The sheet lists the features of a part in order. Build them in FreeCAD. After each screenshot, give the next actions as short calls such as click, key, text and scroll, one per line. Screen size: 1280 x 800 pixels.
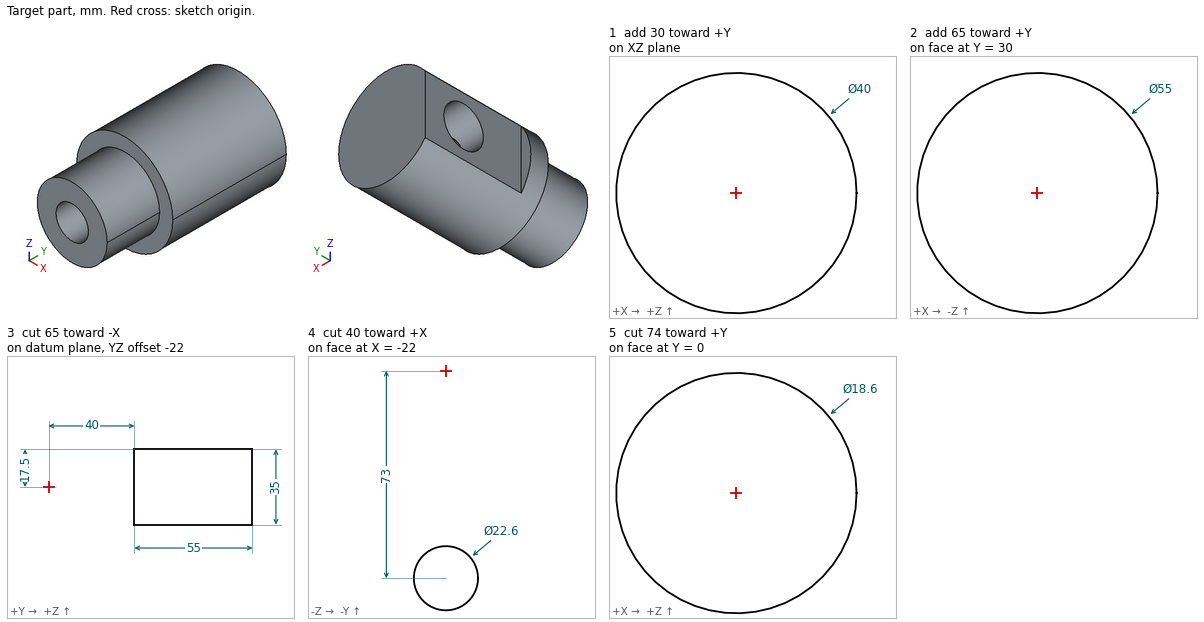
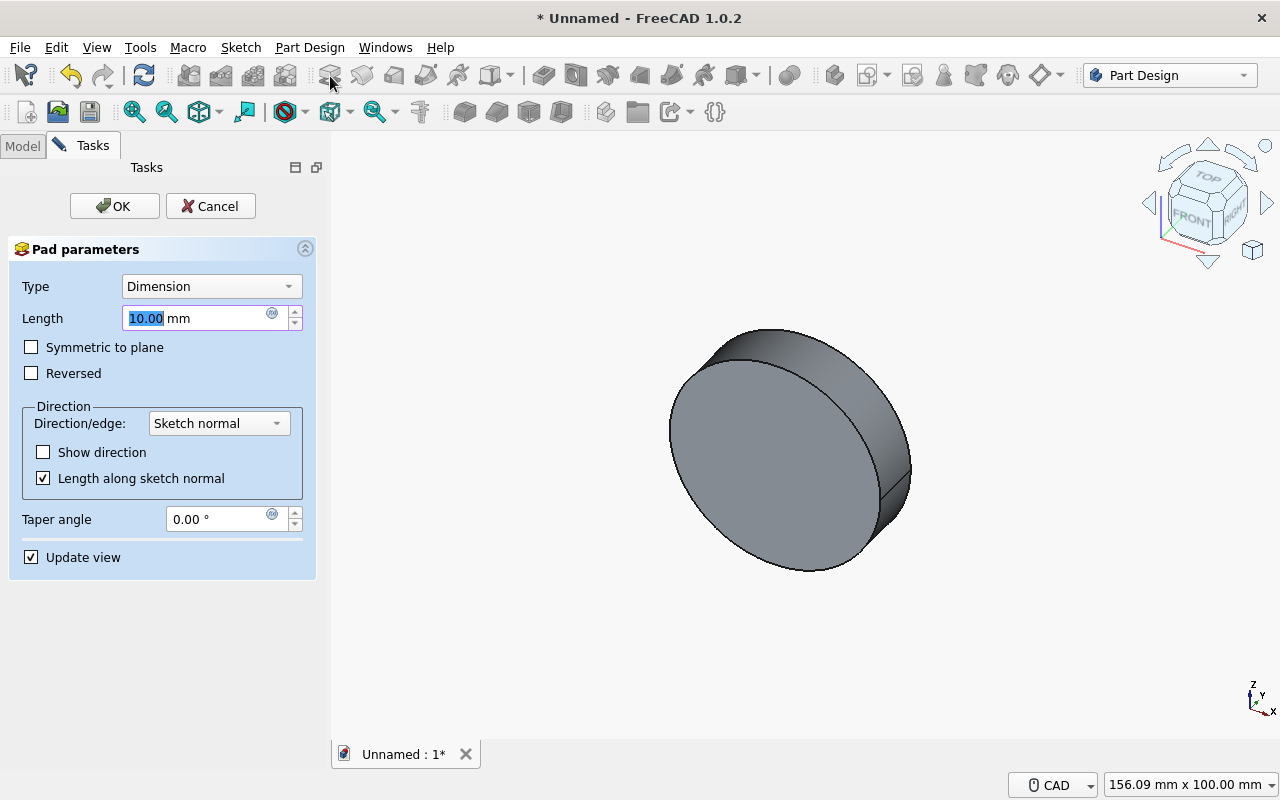
text(30)
key(Tab)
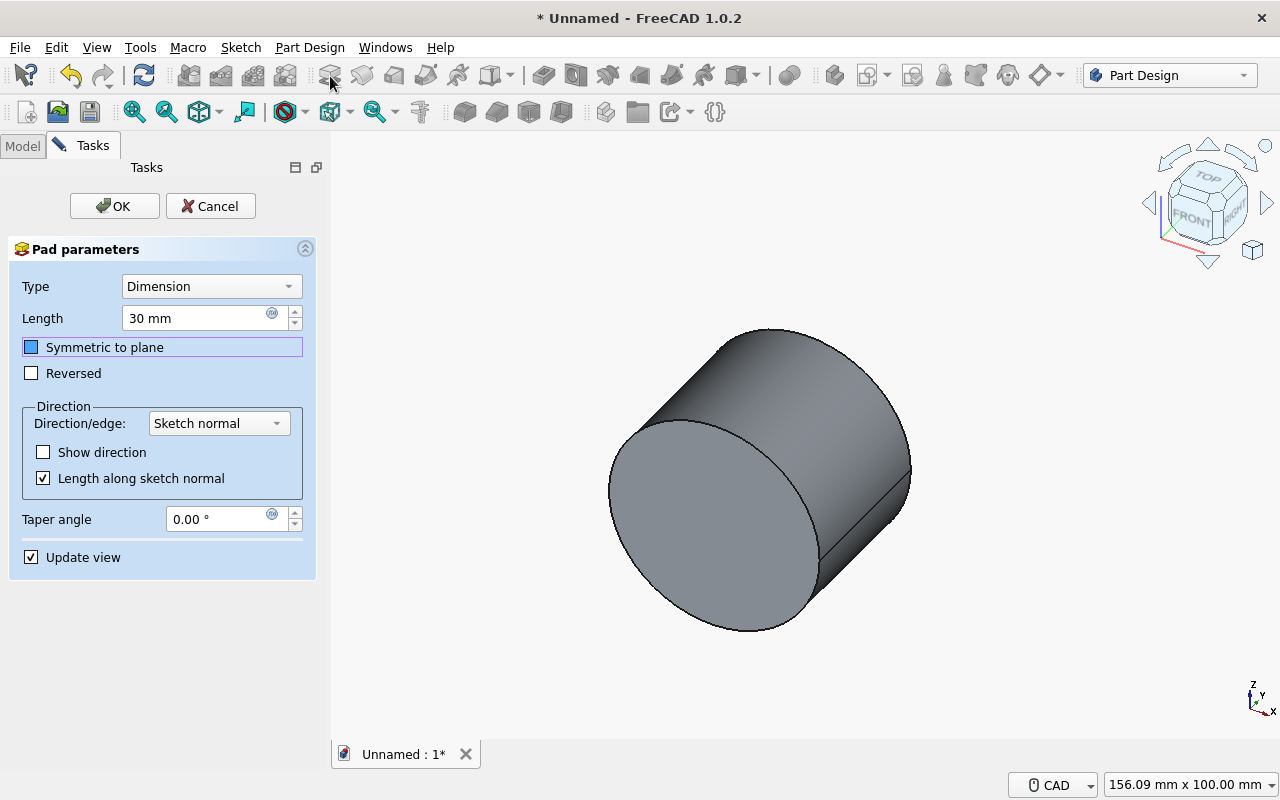
click(30, 373)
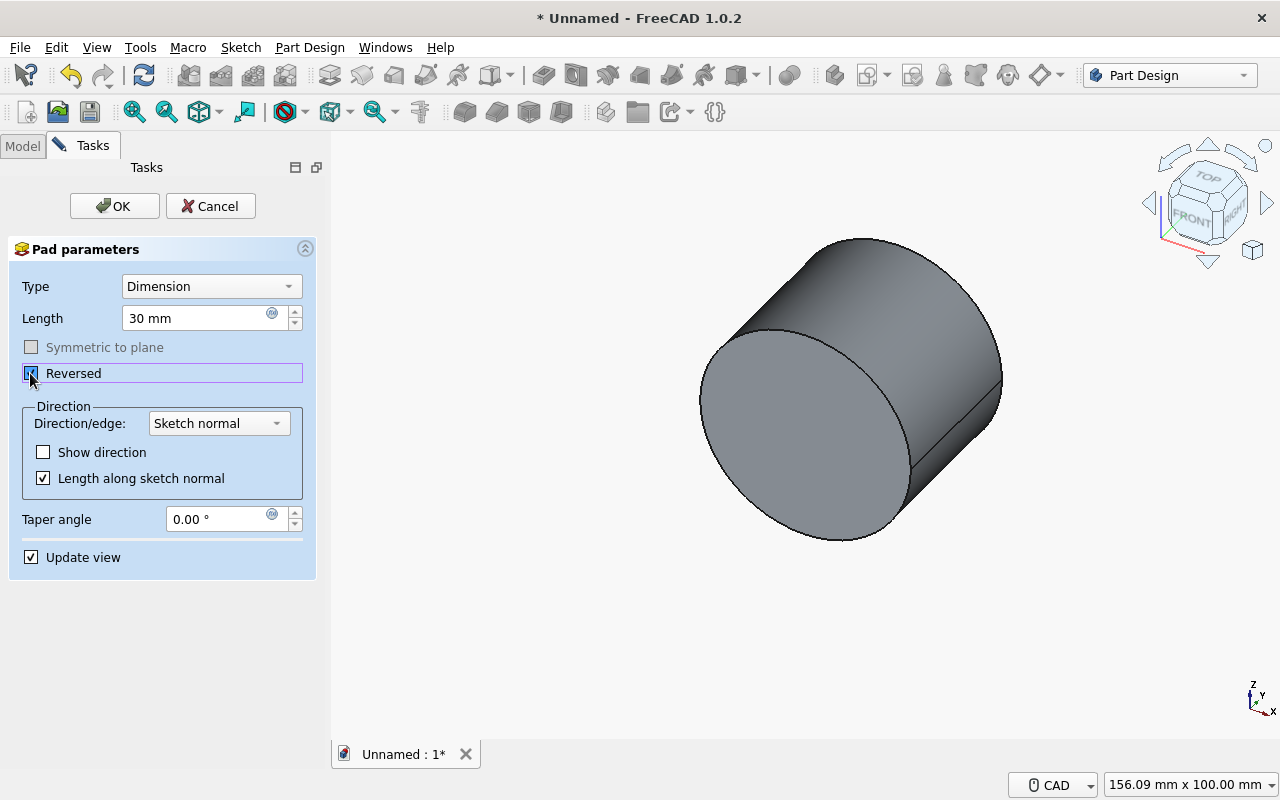
click(115, 206)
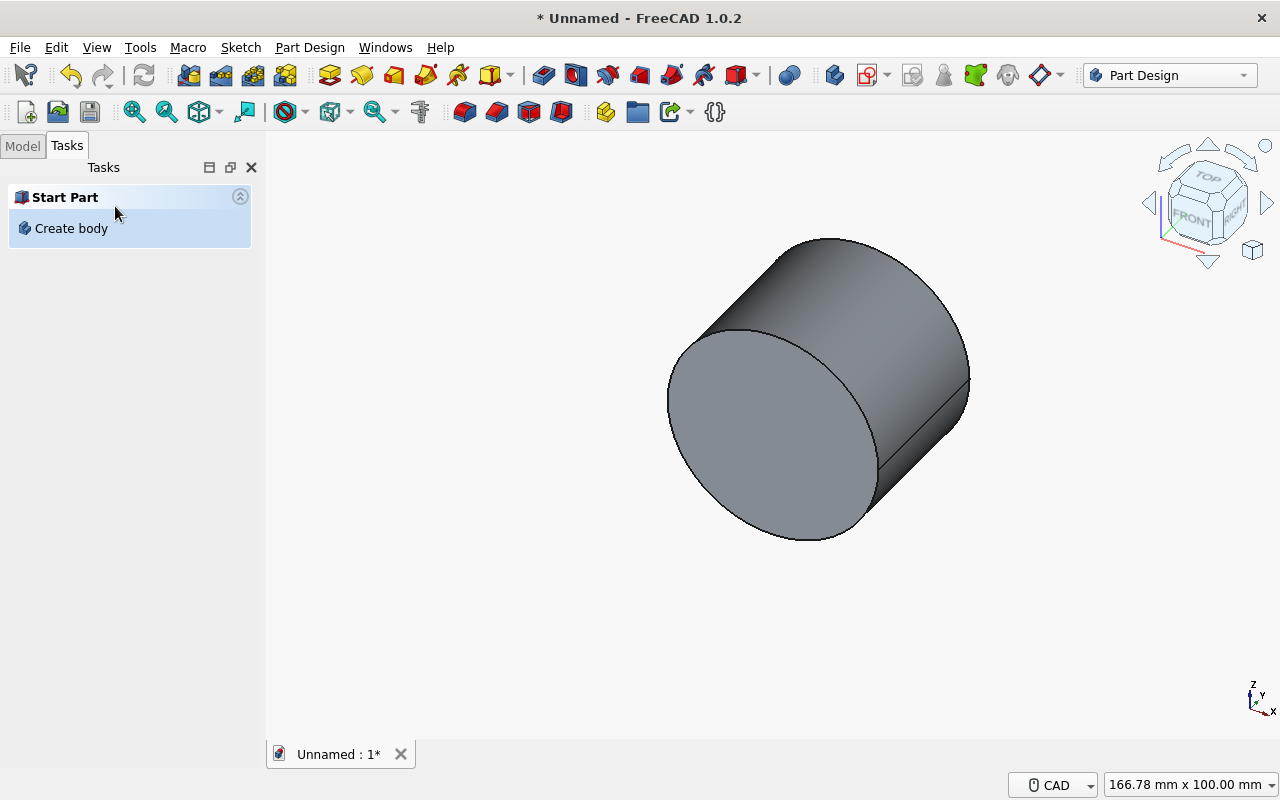
key(4)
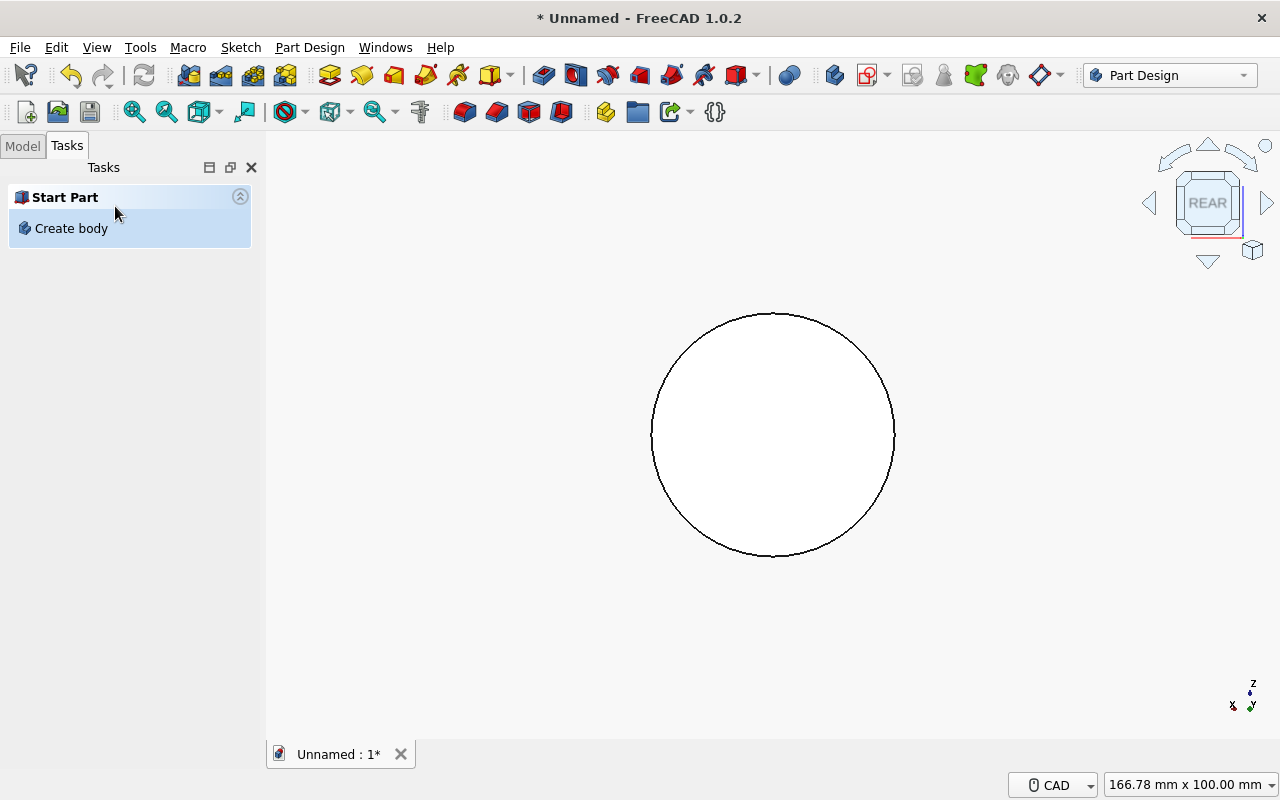
click(136, 112)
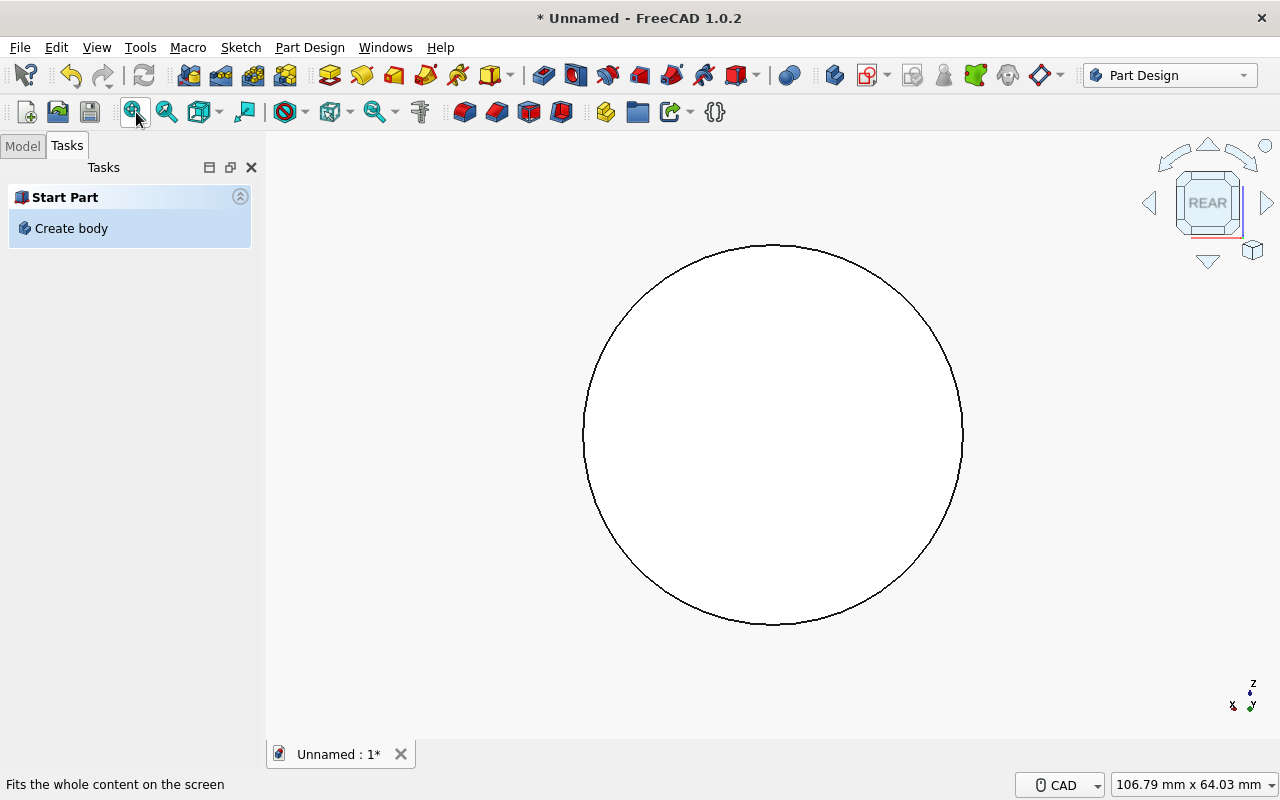
click(773, 434)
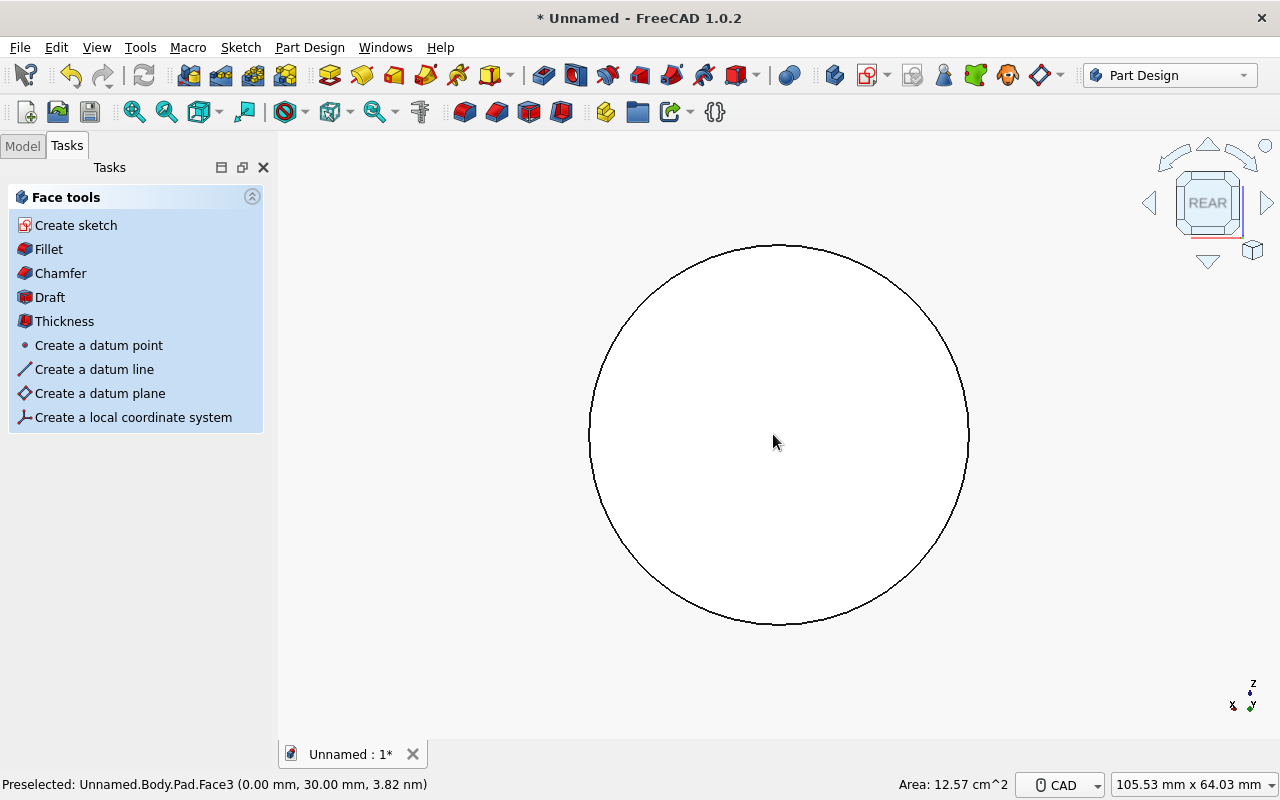
click(868, 76)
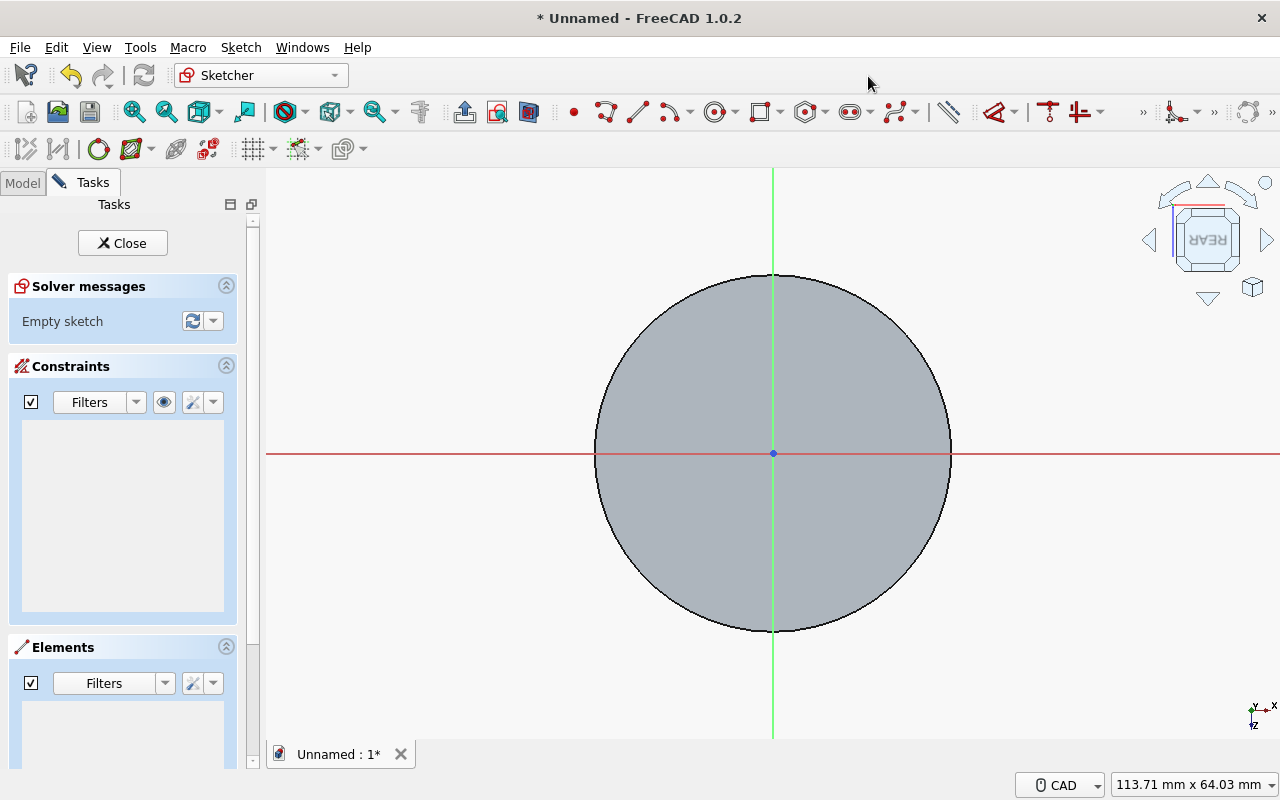
scroll(395, 454, down, 1)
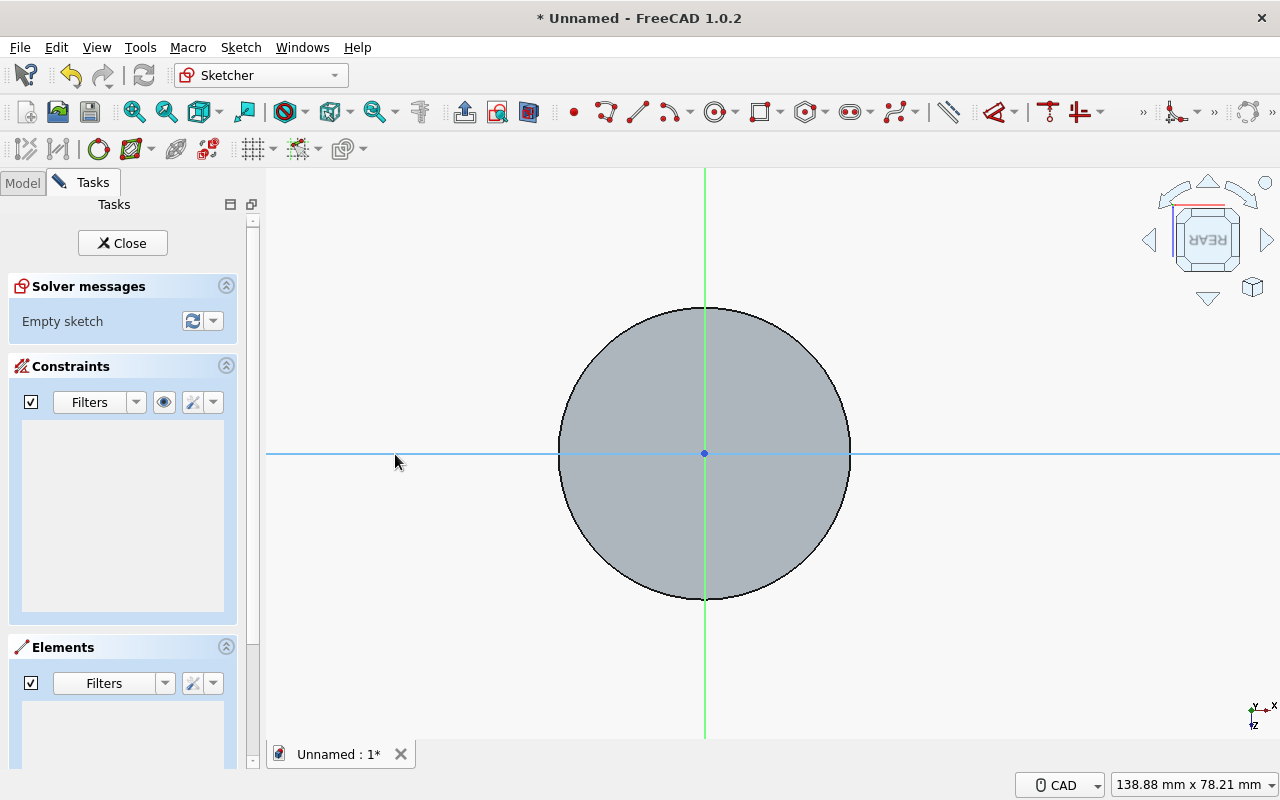
key(g)
key(c)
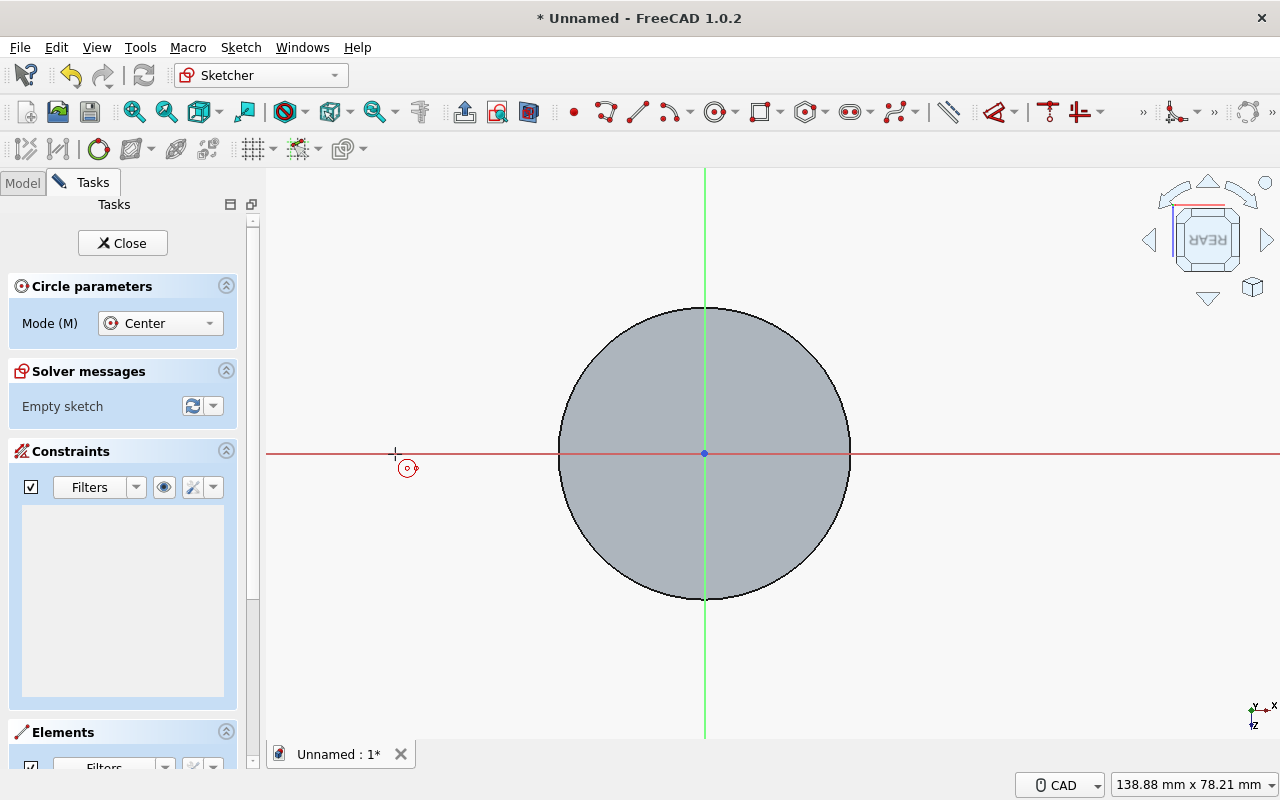
click(705, 454)
move(846, 312)